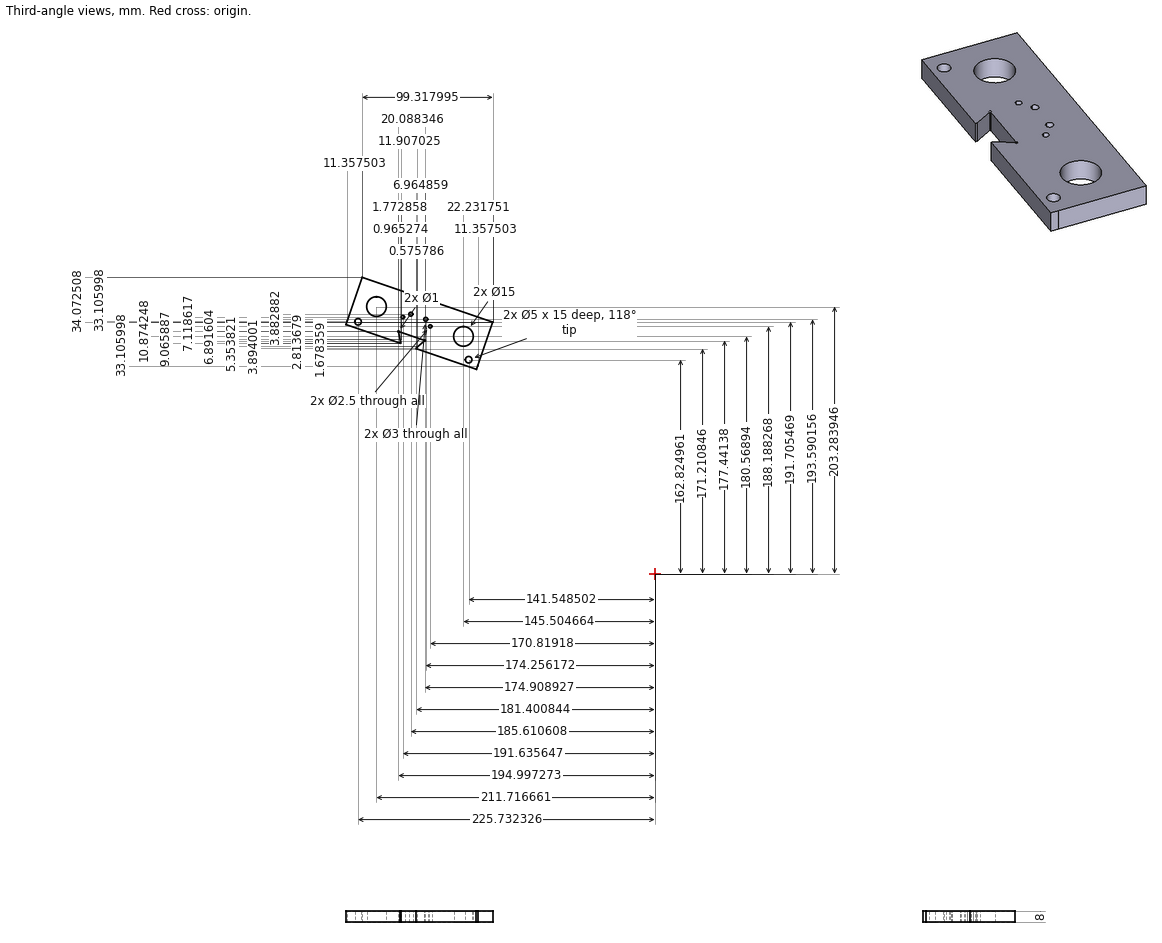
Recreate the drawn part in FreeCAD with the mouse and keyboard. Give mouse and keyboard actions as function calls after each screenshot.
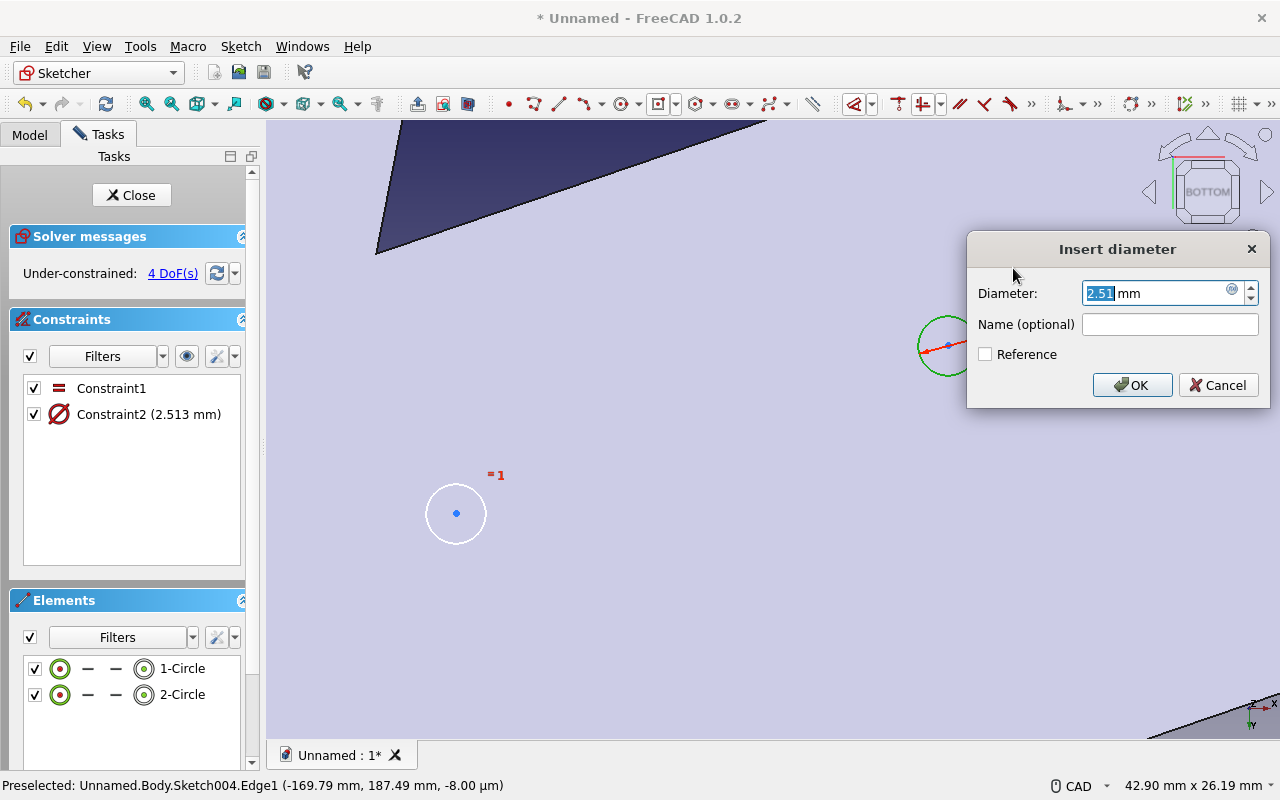
text(2.5)
key(Return)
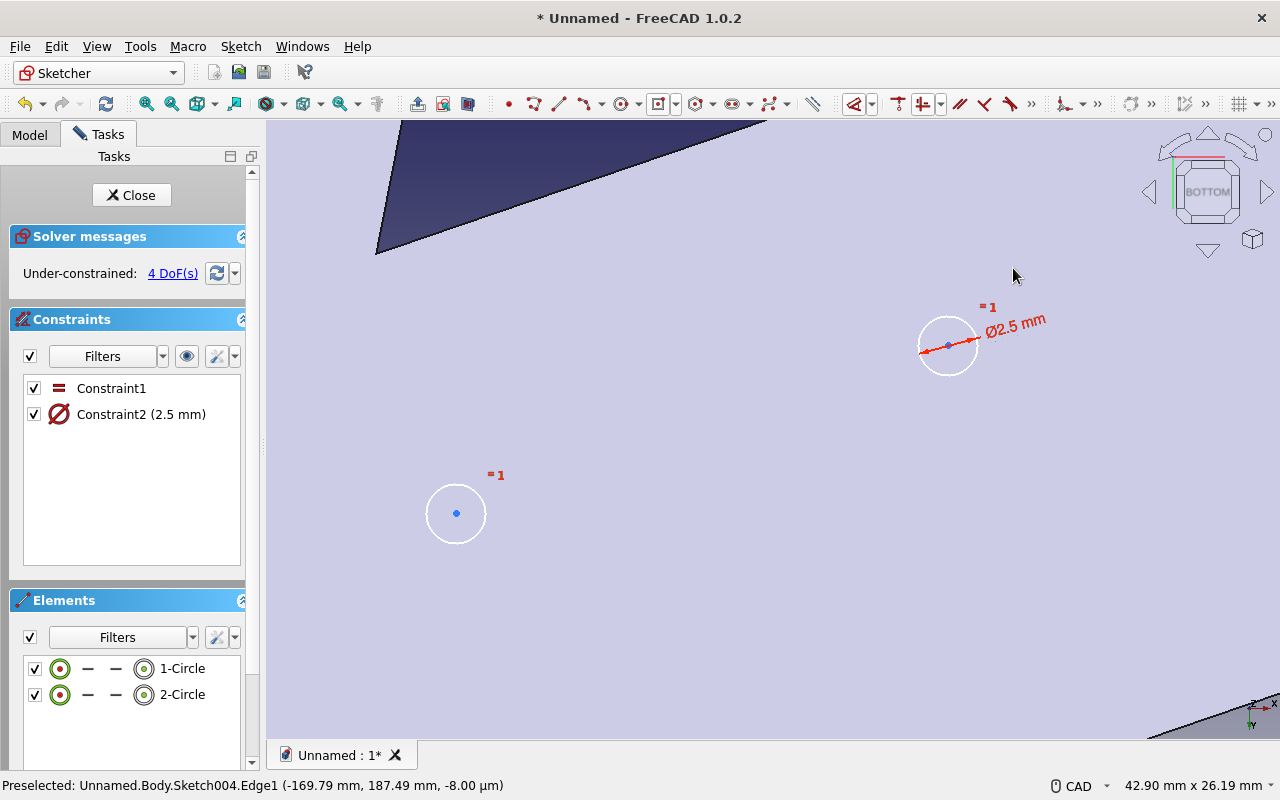
click(948, 346)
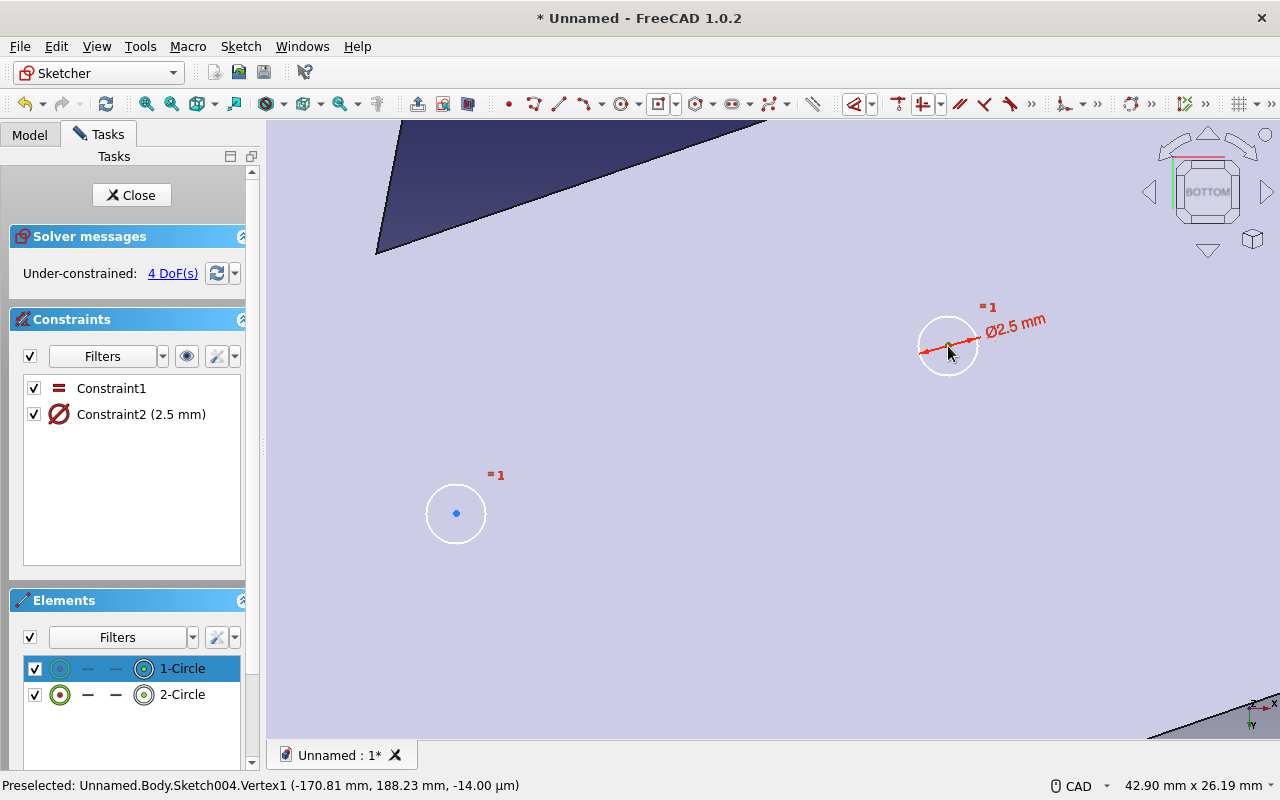
key(l)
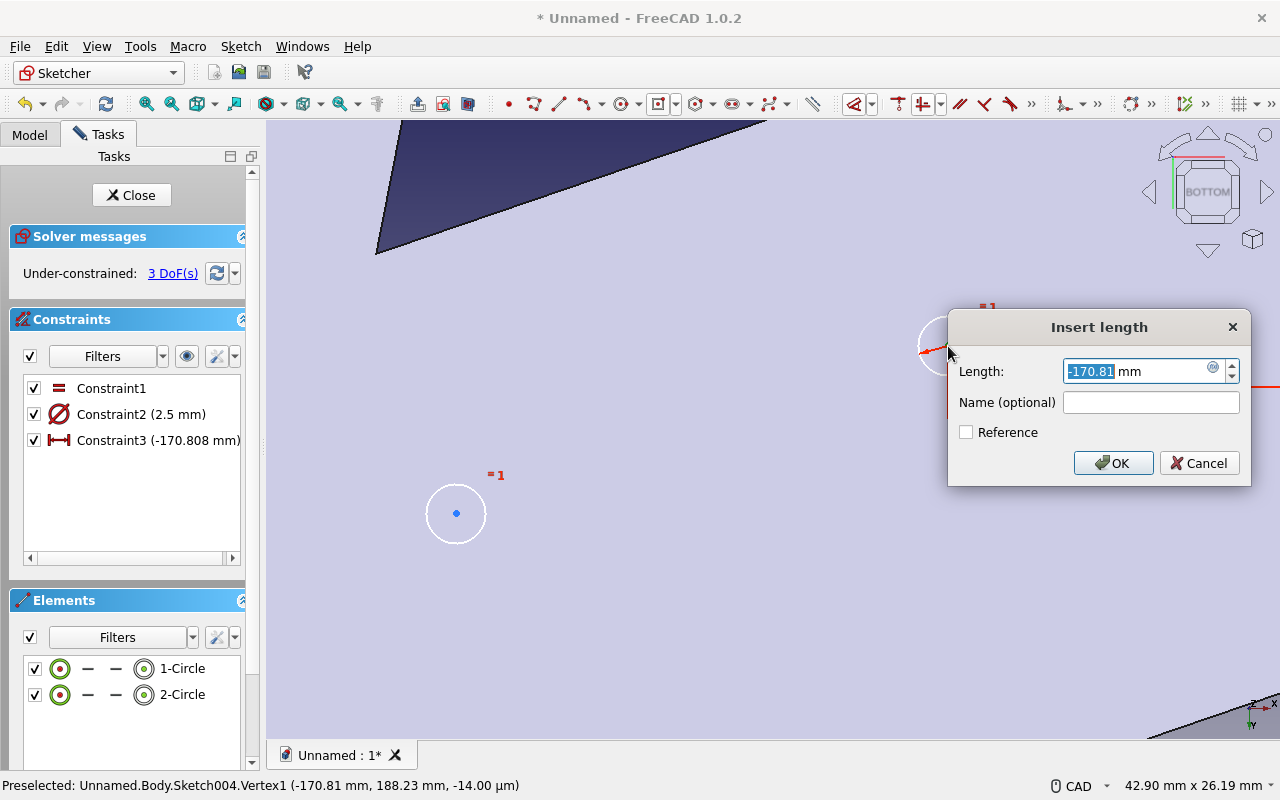
text(-170.81918)
key(Return)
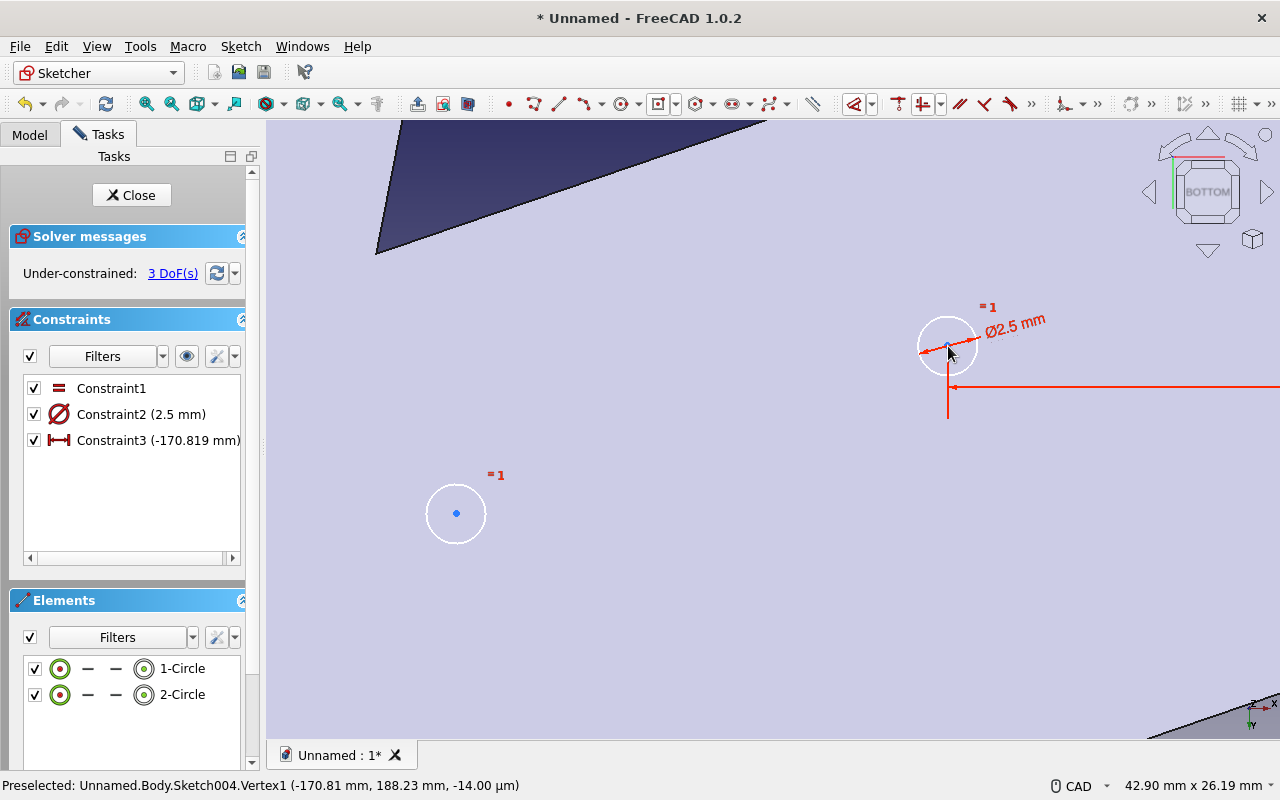
click(948, 346)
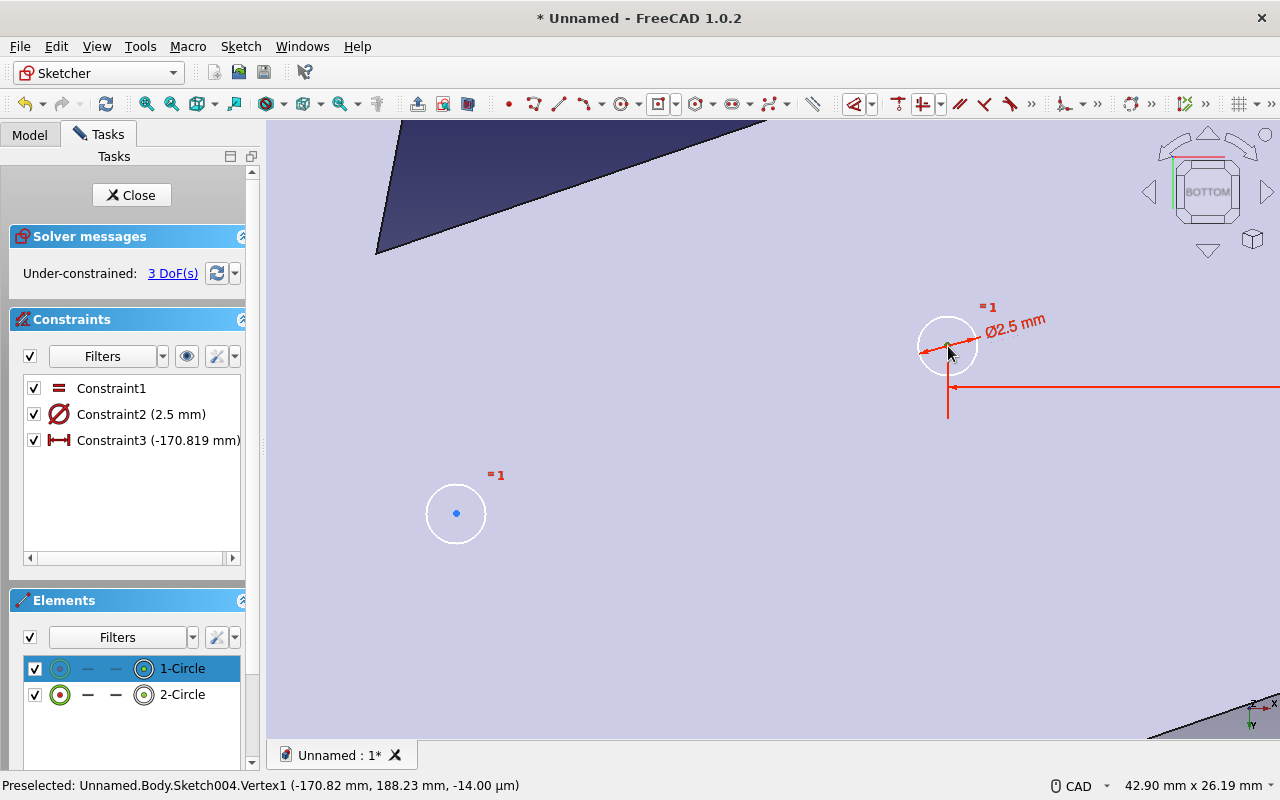
click(456, 514)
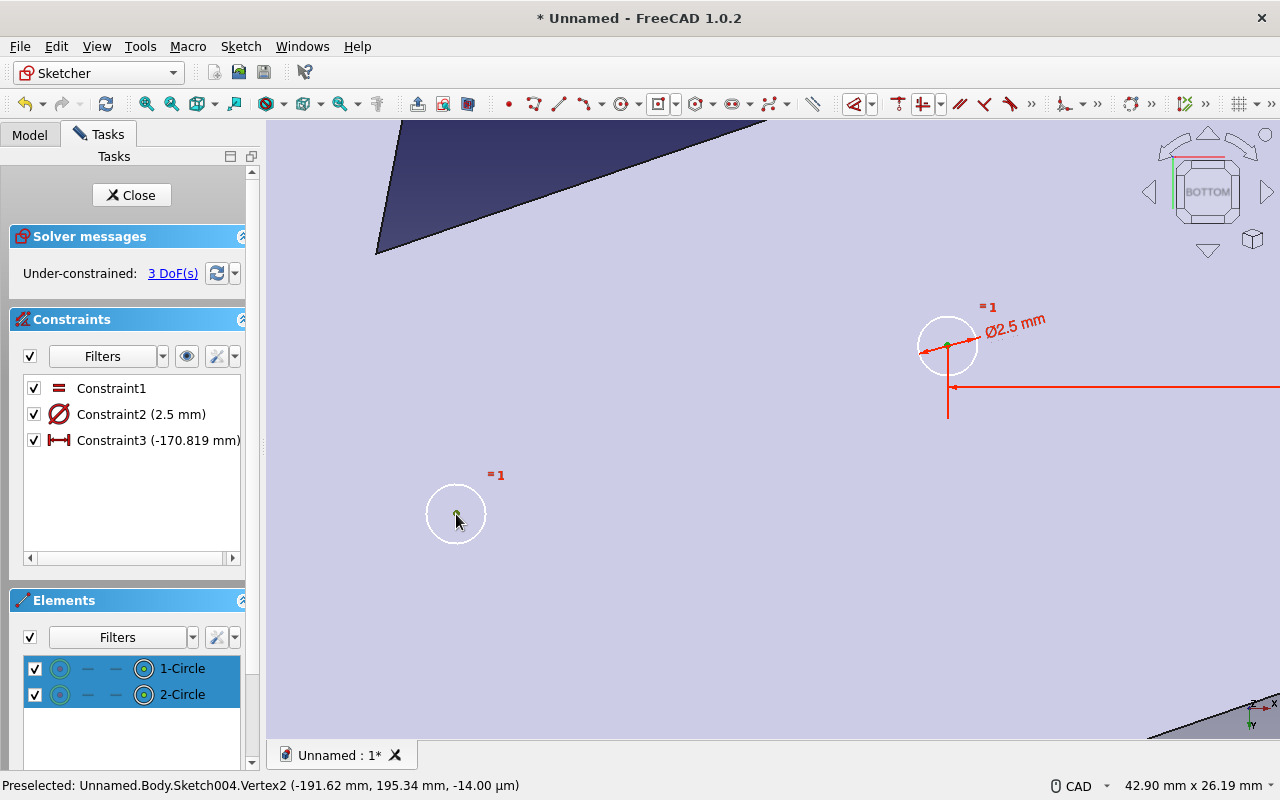
click(872, 104)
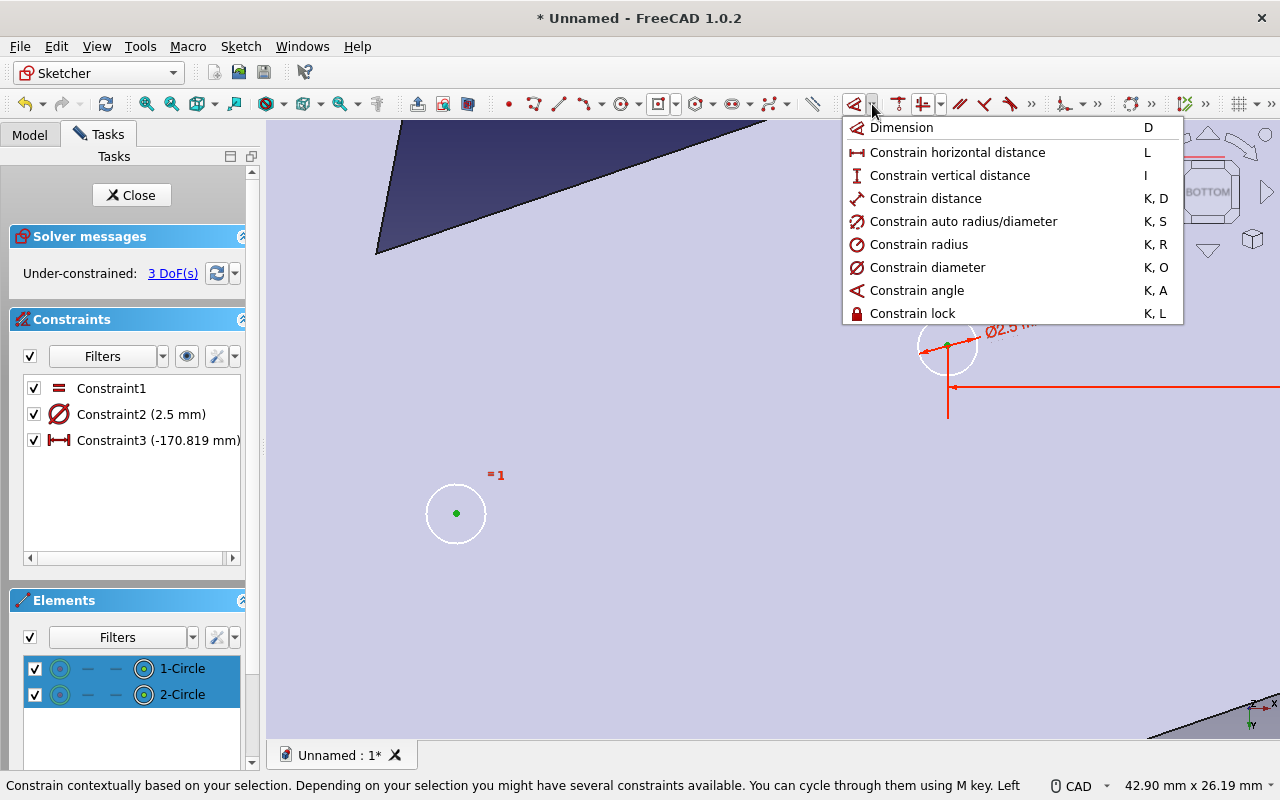
click(1013, 176)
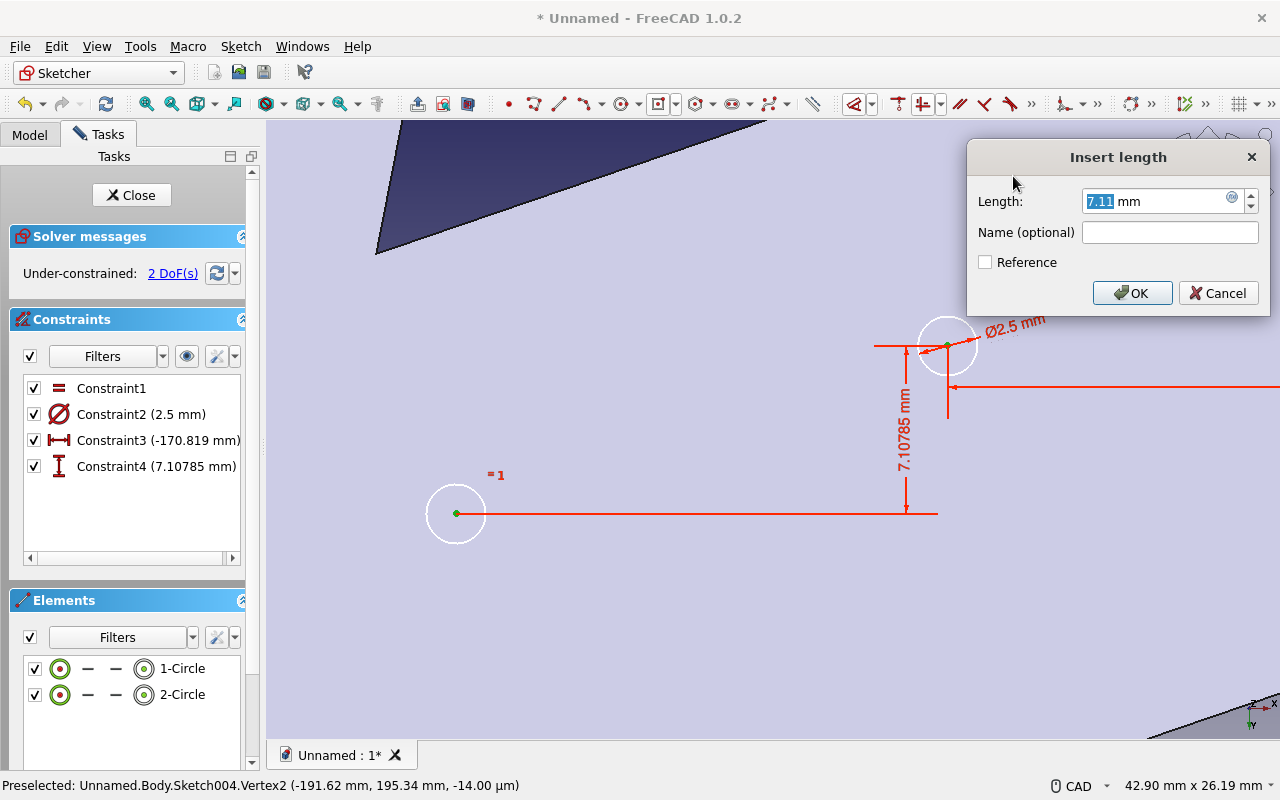
text(7.118617)
key(Return)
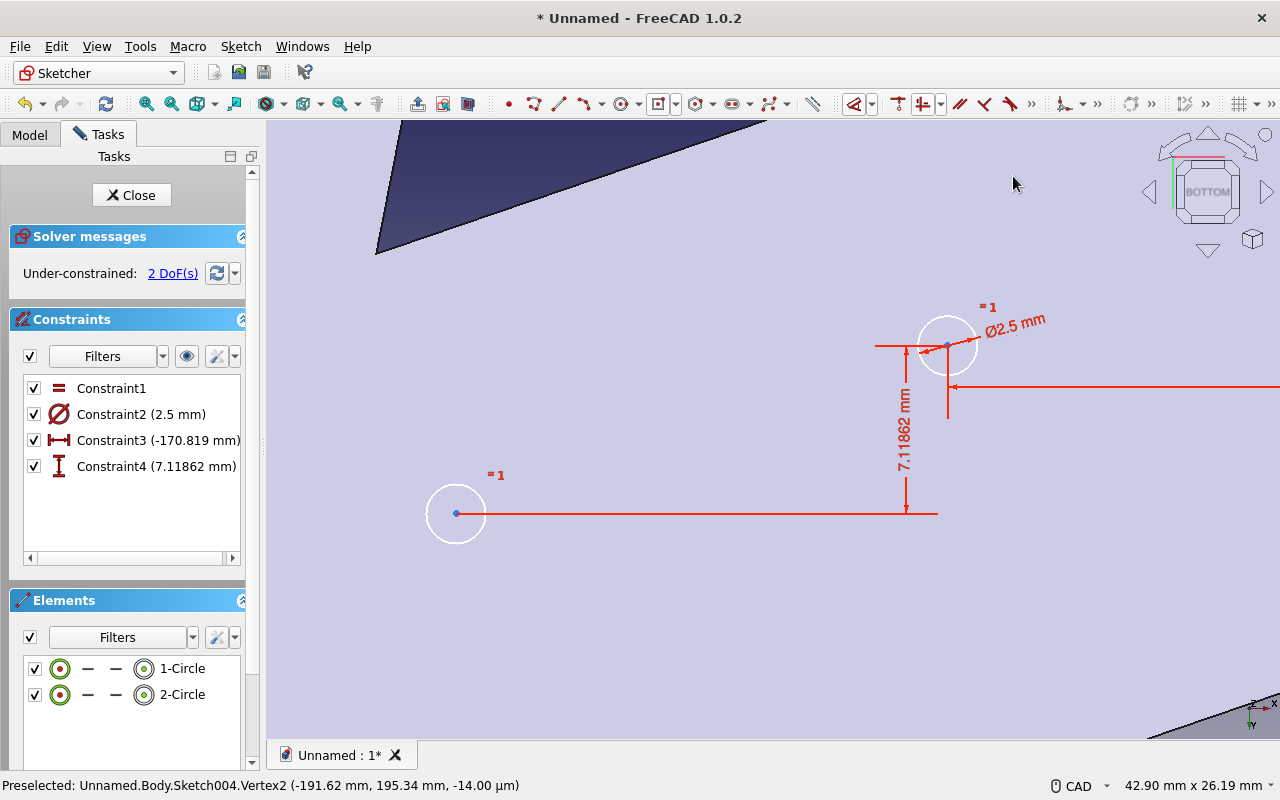
click(948, 346)